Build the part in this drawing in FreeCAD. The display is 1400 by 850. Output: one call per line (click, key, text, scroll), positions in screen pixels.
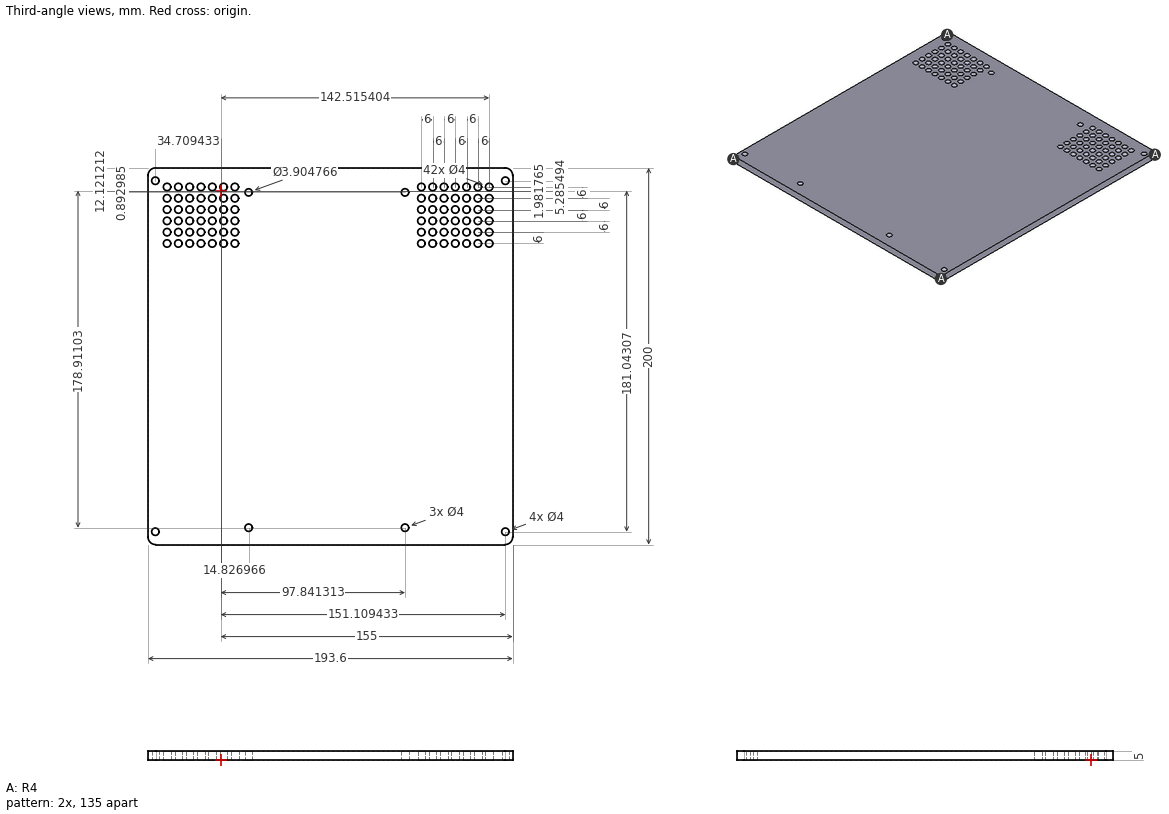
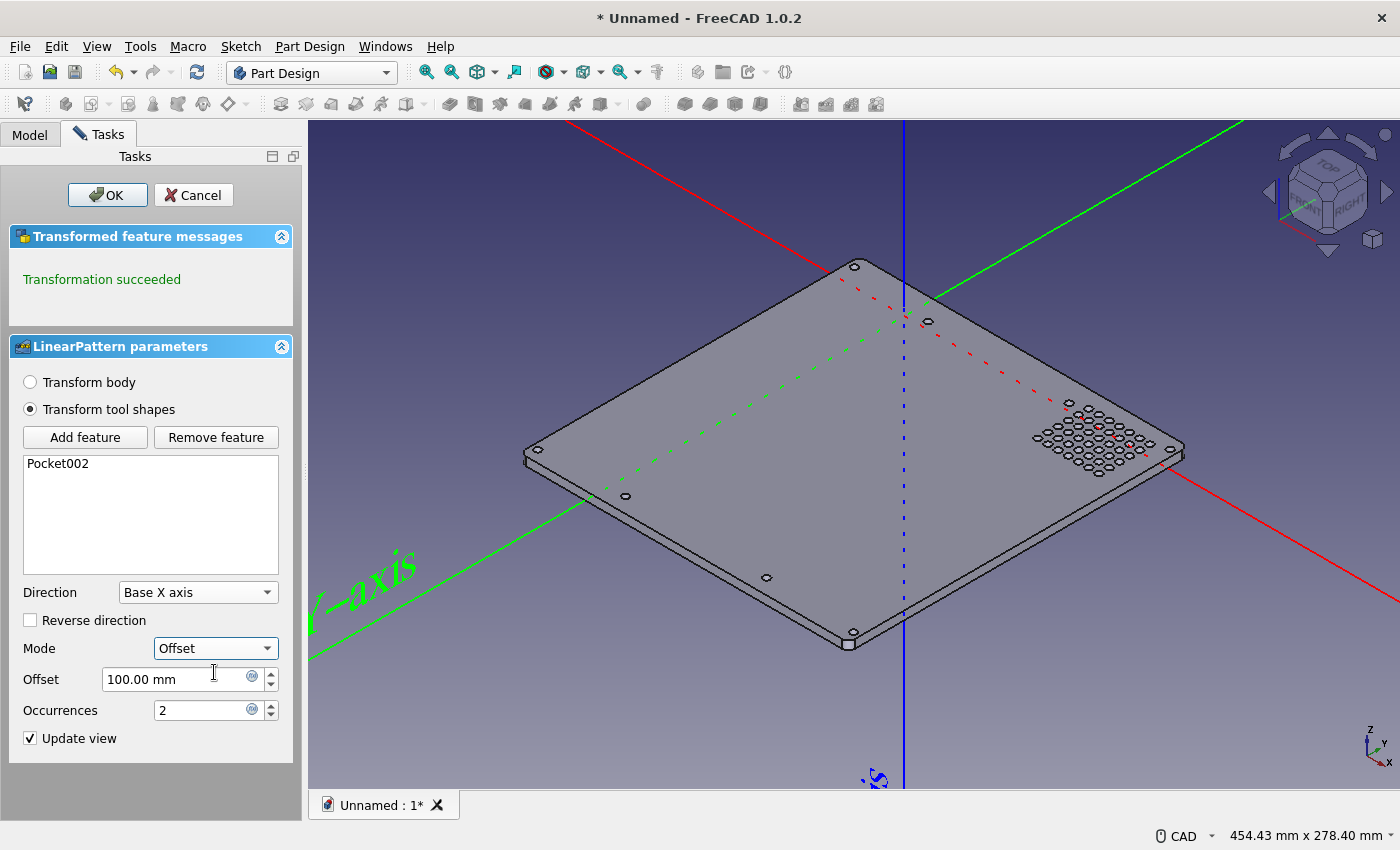
triple_click(184, 680)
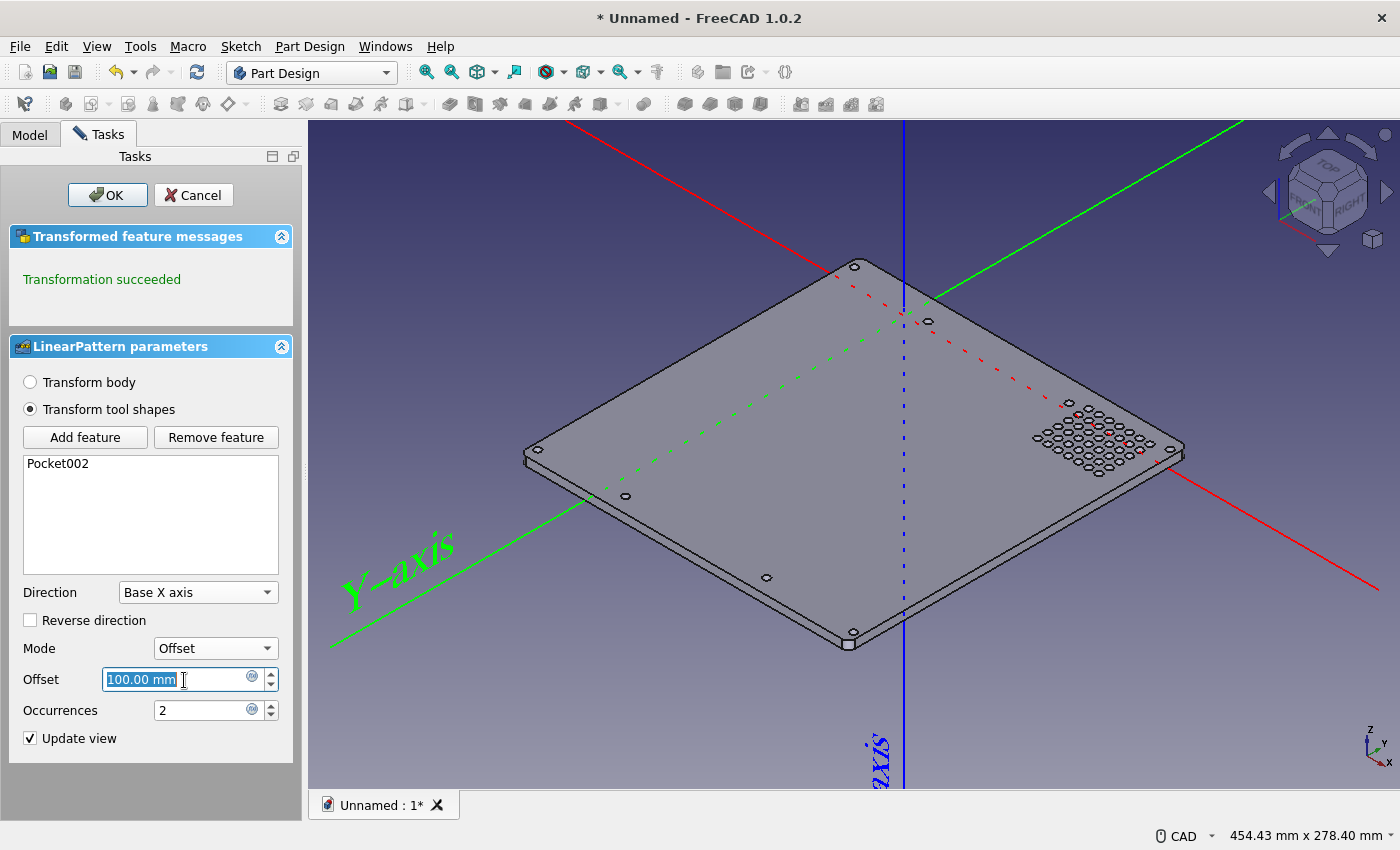
text(135)
key(Tab)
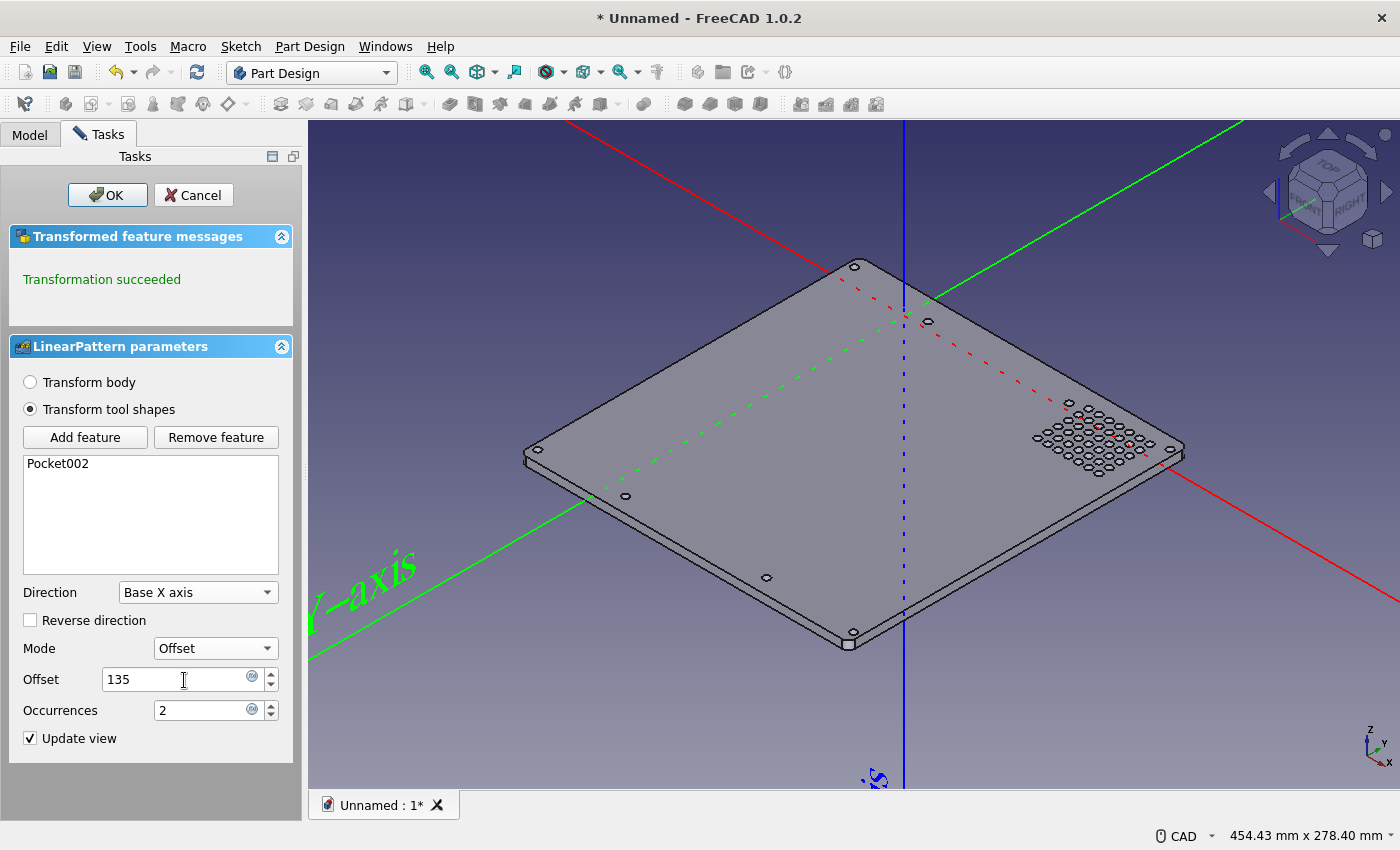
triple_click(210, 710)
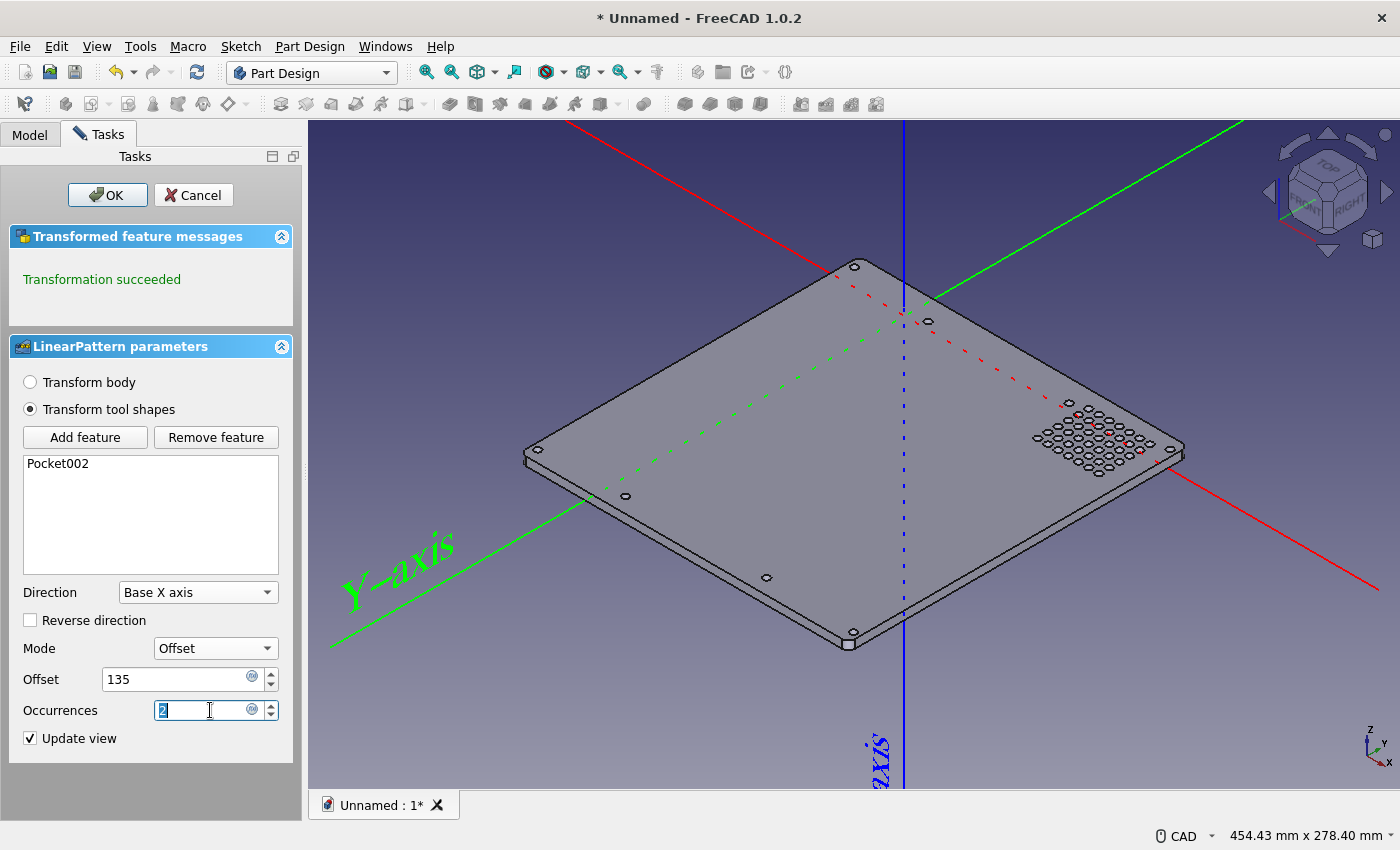
text(2)
key(Tab)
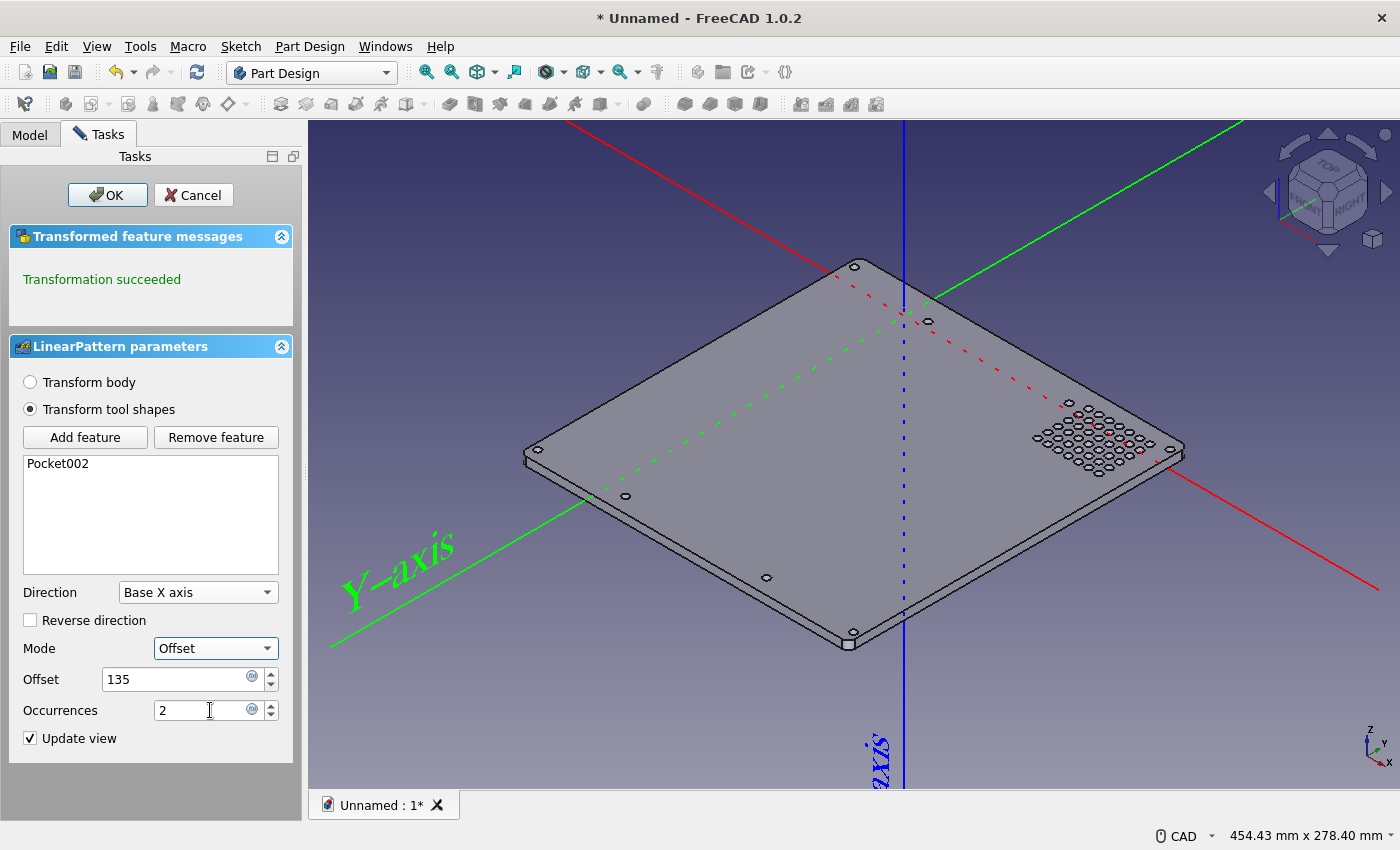
click(31, 620)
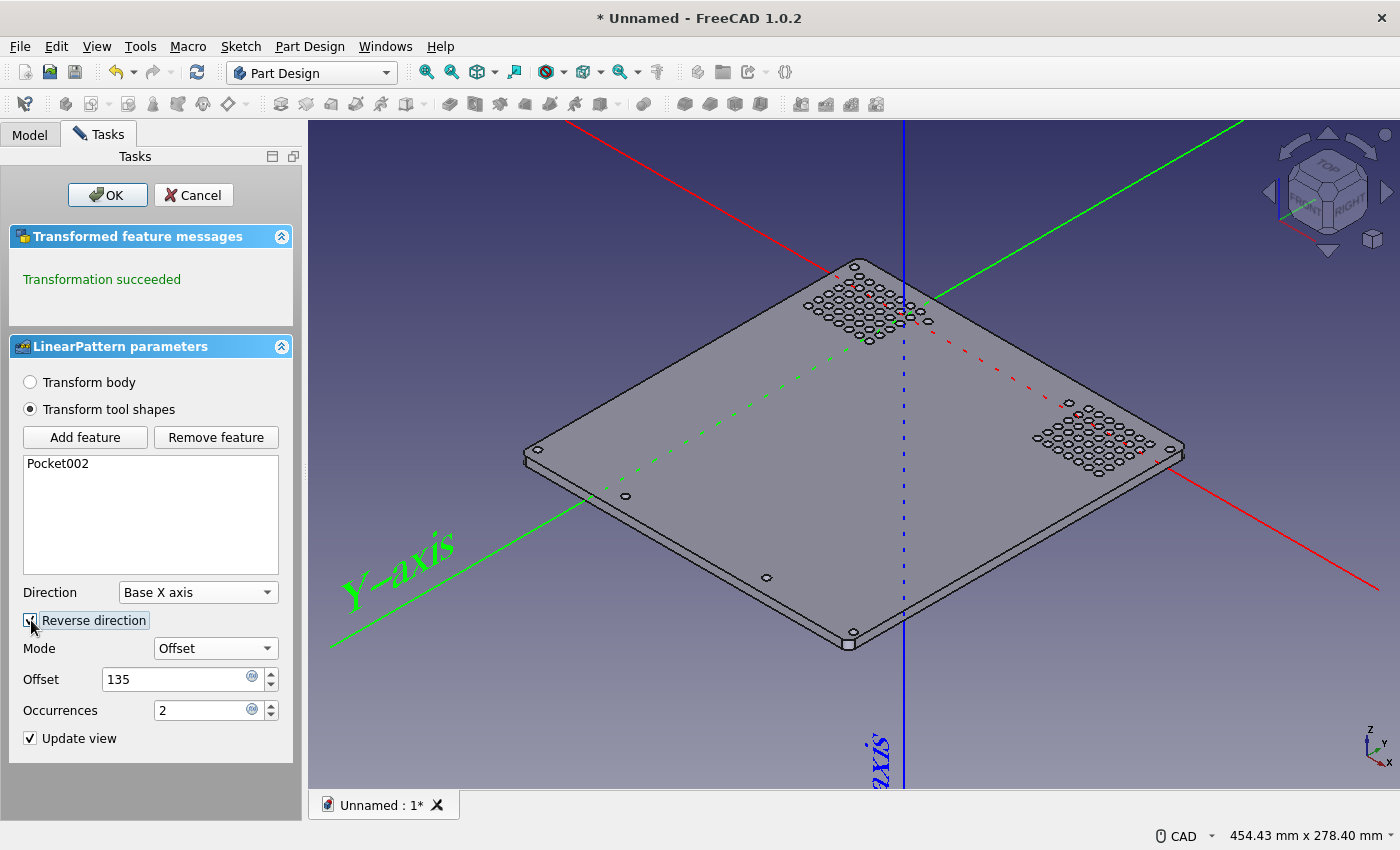
click(108, 195)